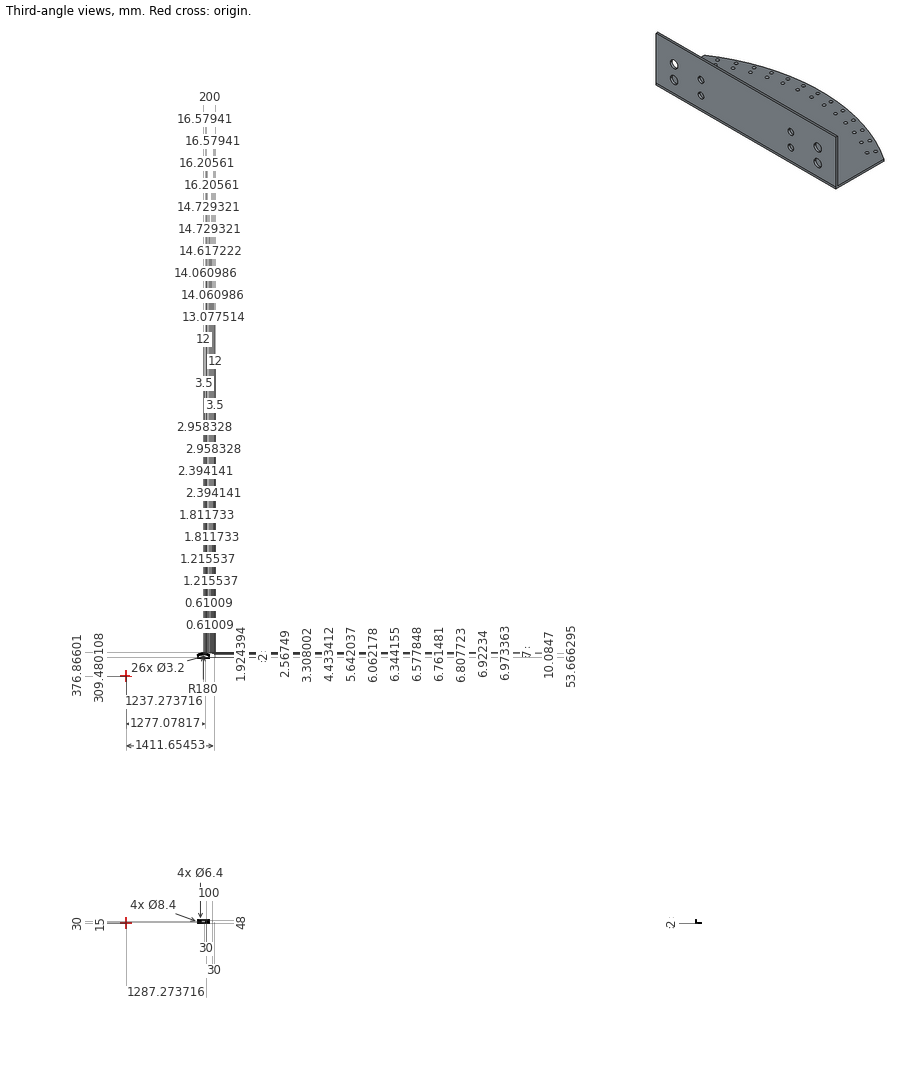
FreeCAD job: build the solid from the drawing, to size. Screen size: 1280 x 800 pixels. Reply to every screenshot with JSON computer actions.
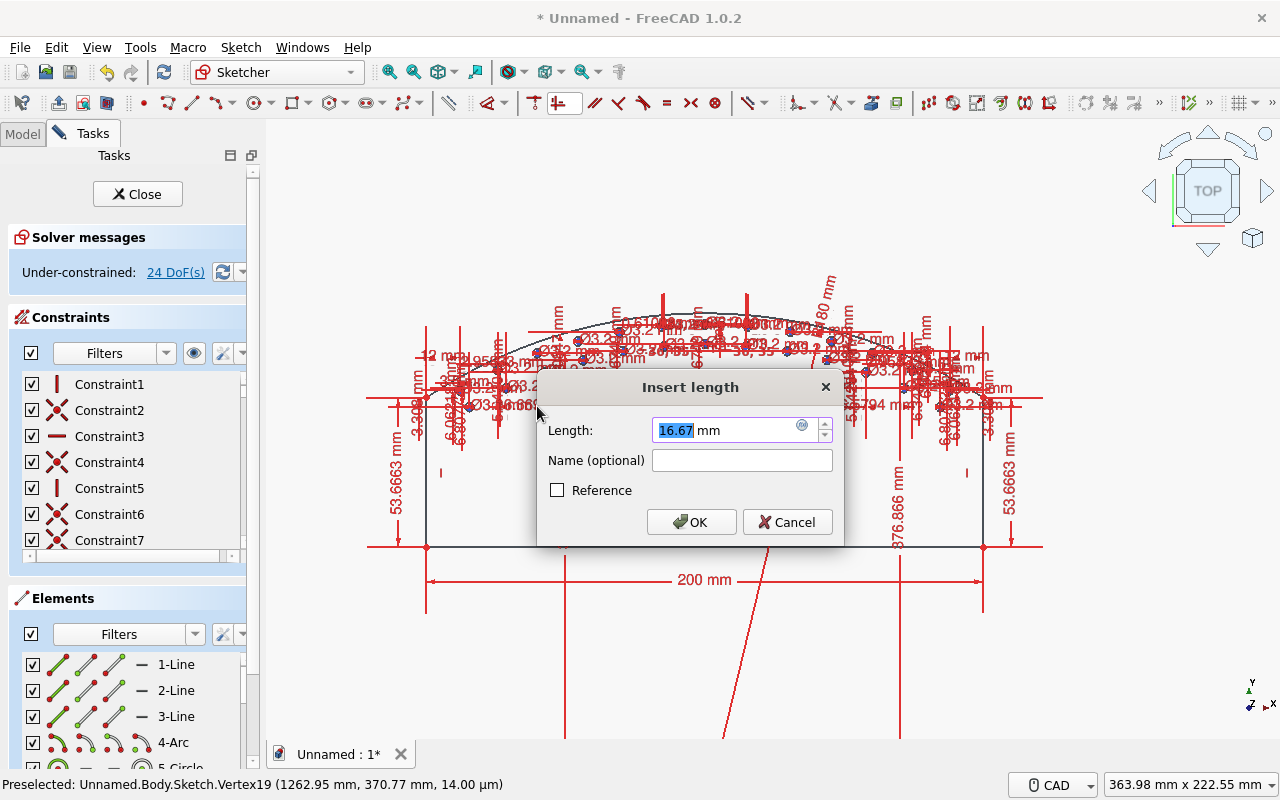
{"action": "type", "text": "16.57941"}
{"action": "key", "text": "Return"}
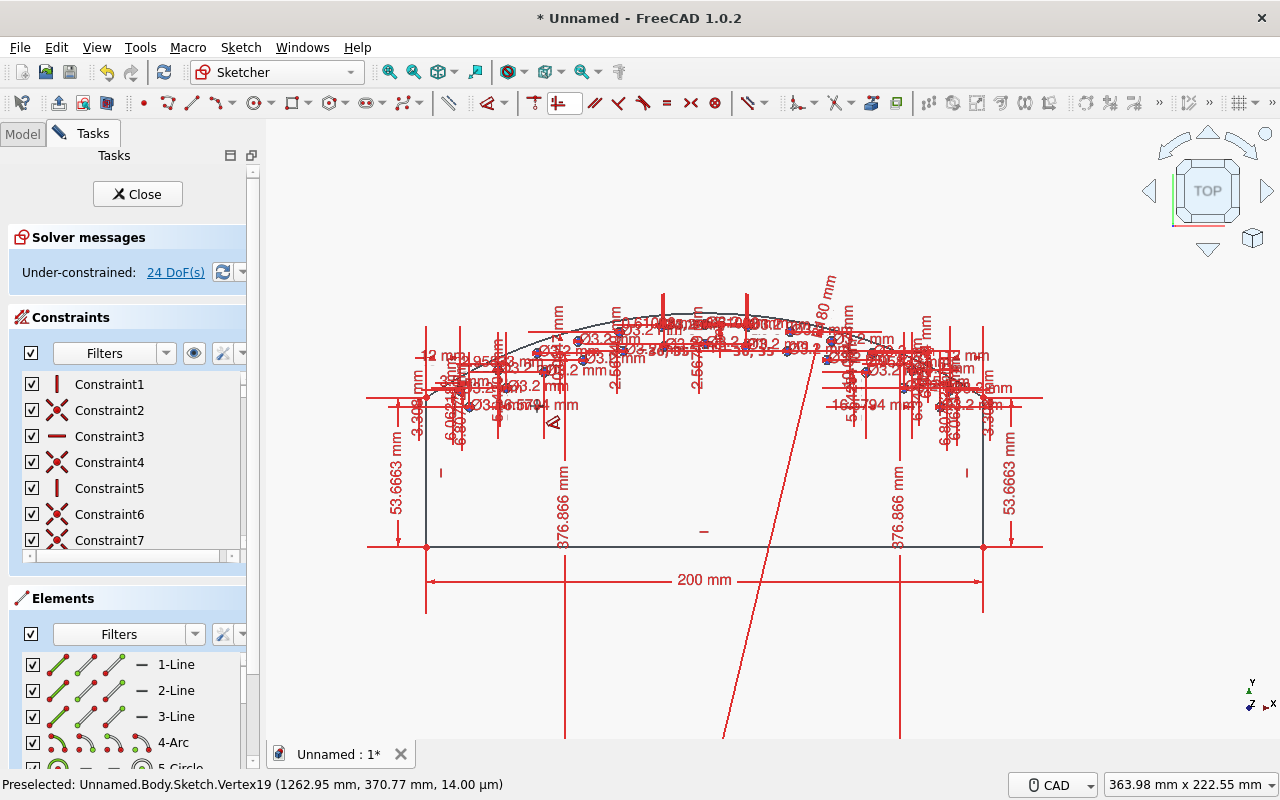
{"action": "scroll", "coordinate": [506, 388], "scroll_direction": "up", "scroll_amount": 5}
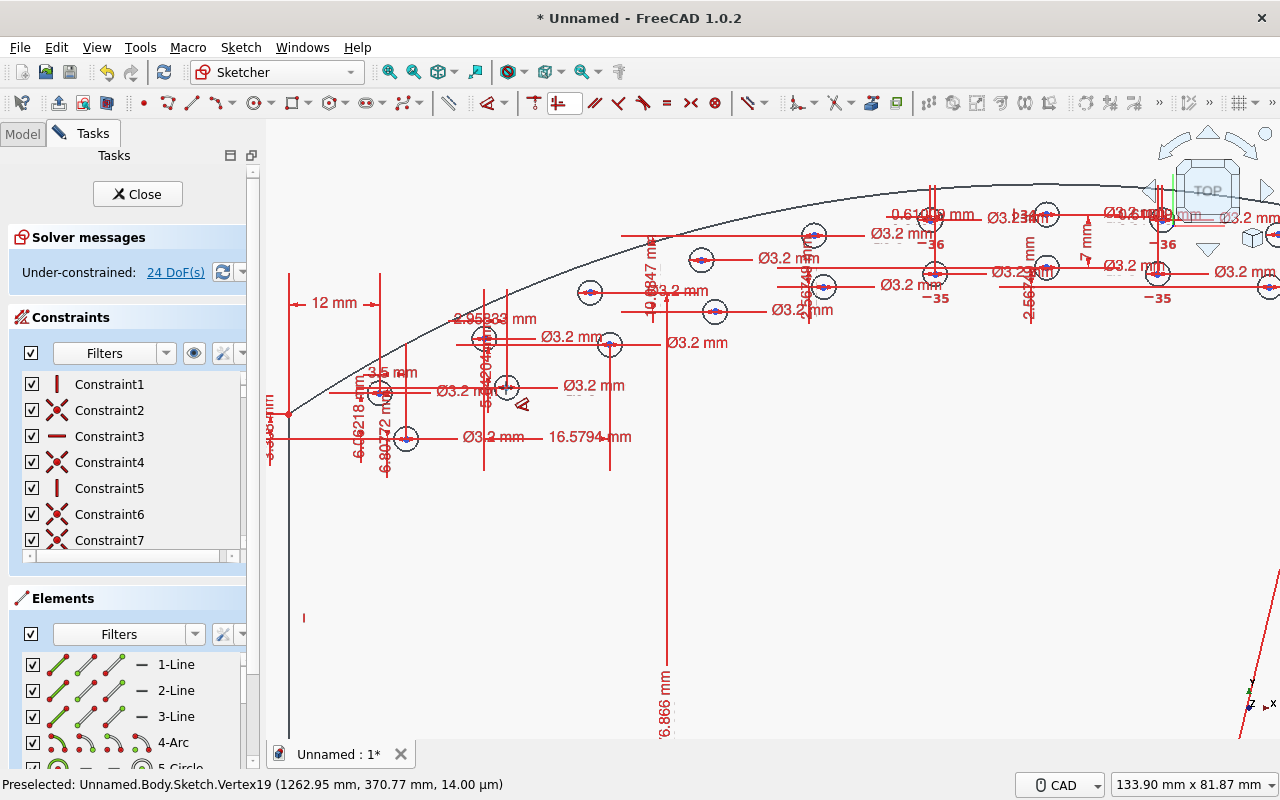
{"action": "left_click", "coordinate": [507, 388]}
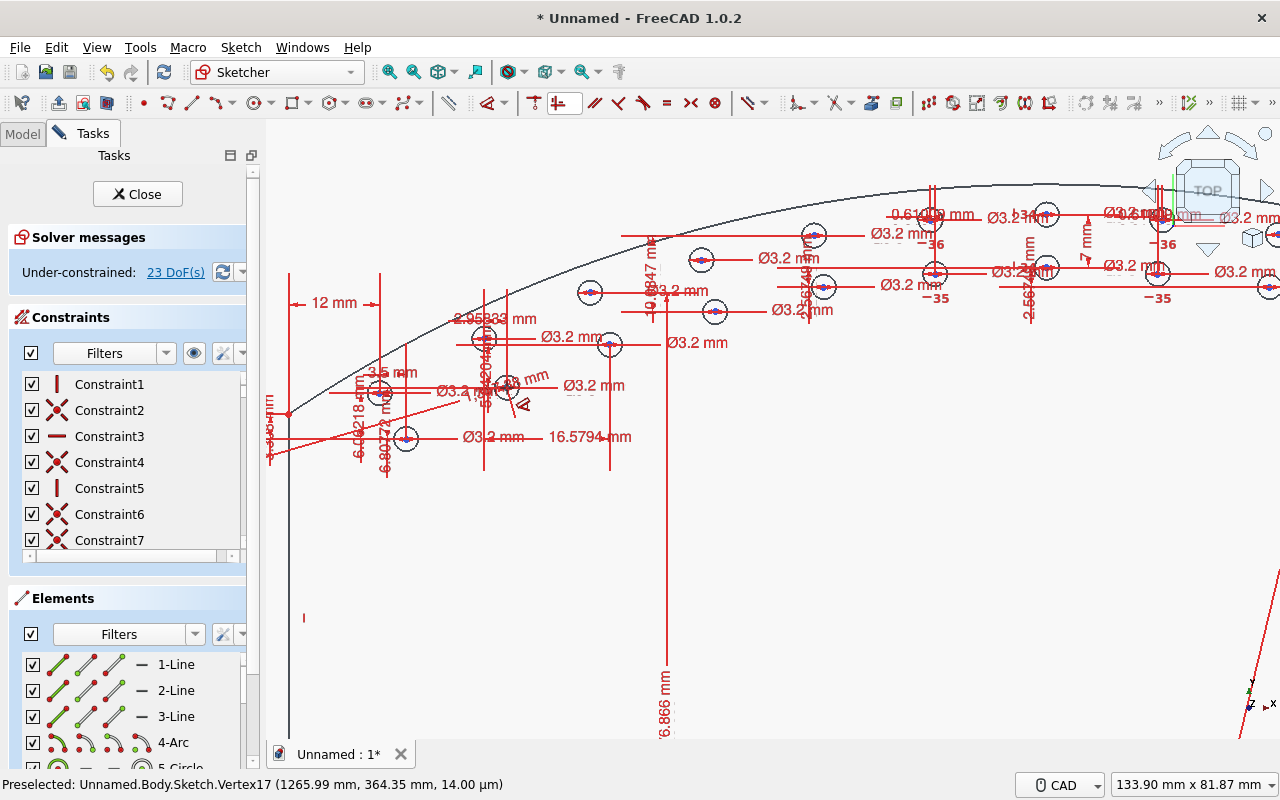
{"action": "left_click", "coordinate": [484, 339]}
{"action": "left_click", "coordinate": [450, 346]}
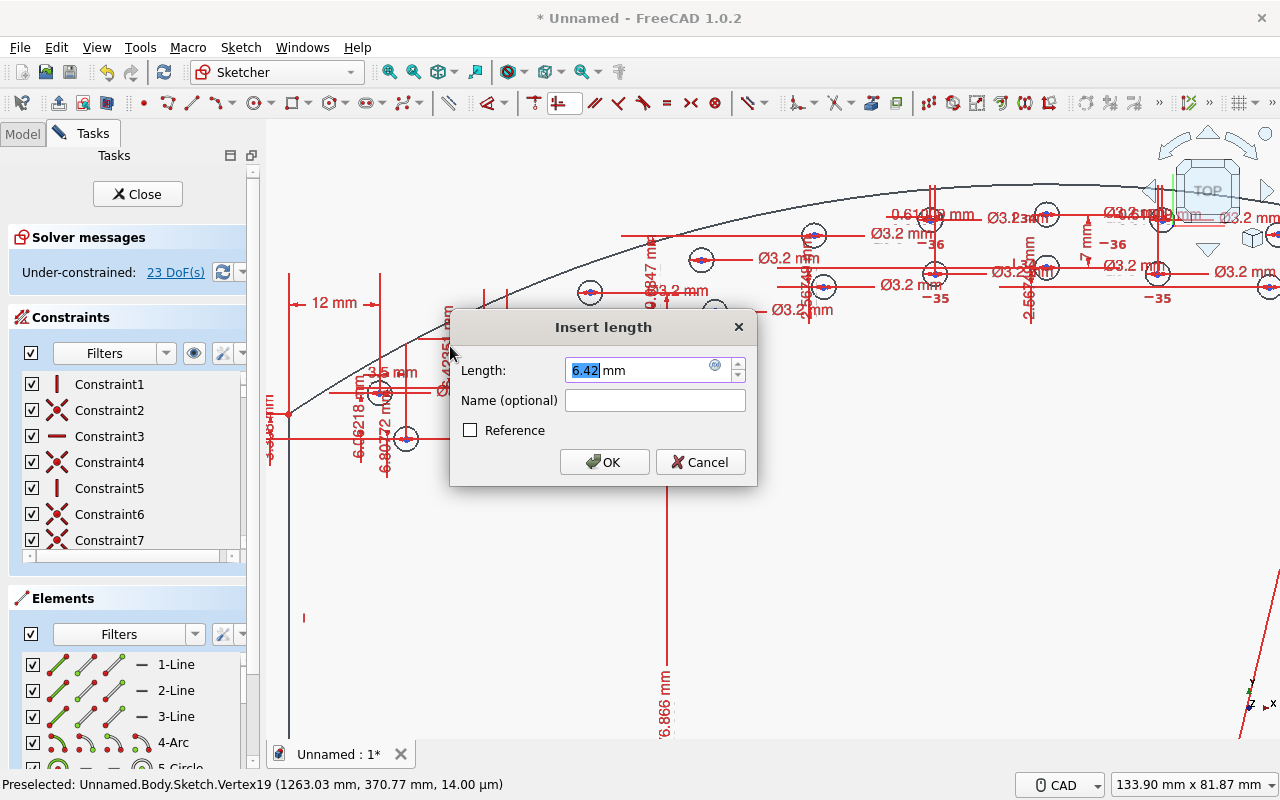
{"action": "type", "text": "6.344155"}
{"action": "key", "text": "Return"}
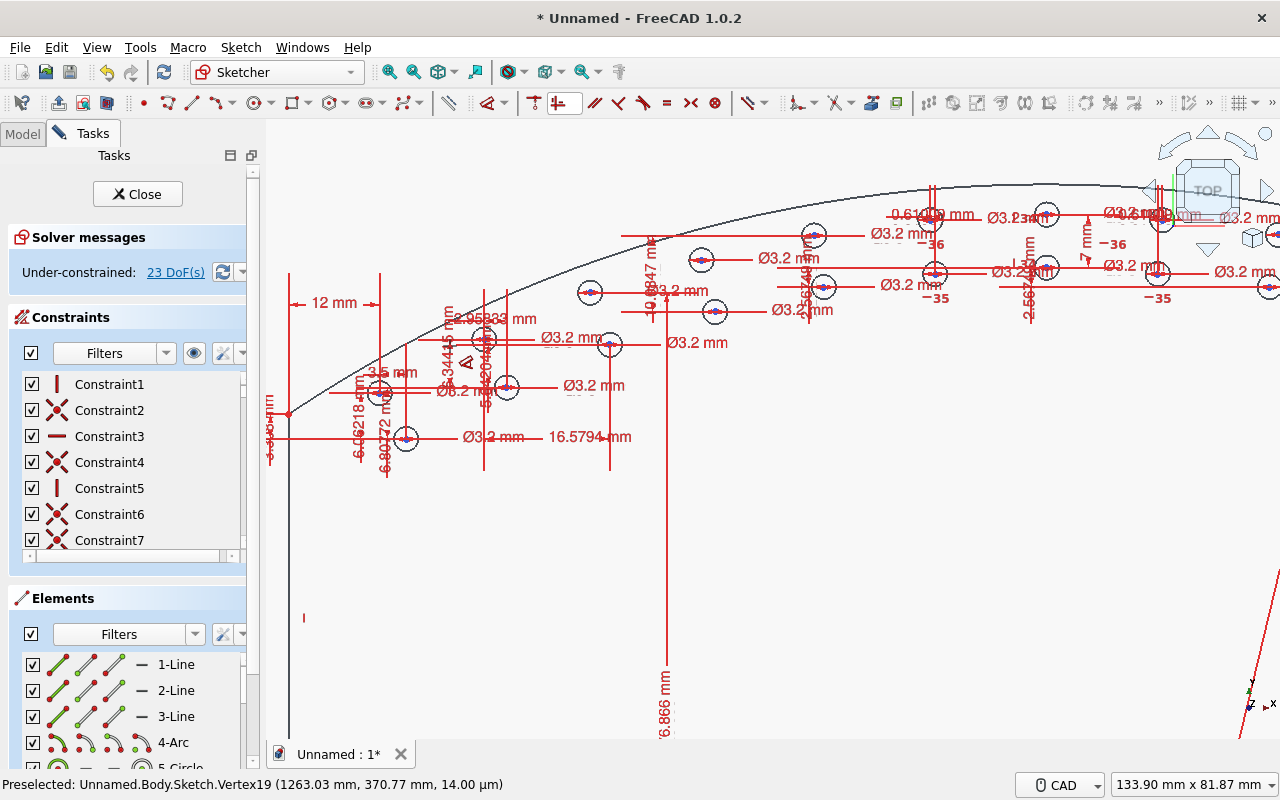
{"action": "scroll", "coordinate": [505, 388], "scroll_direction": "down", "scroll_amount": 5}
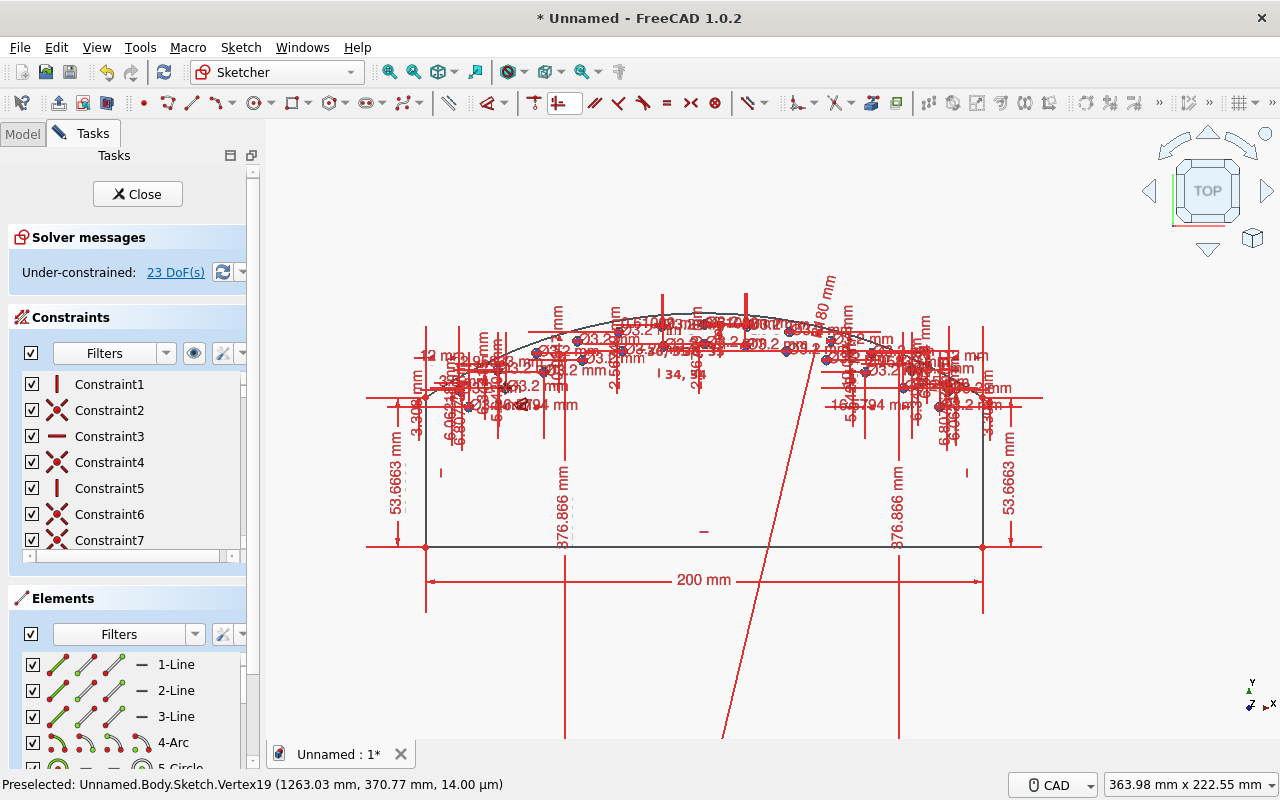
{"action": "scroll", "coordinate": [865, 372], "scroll_direction": "up", "scroll_amount": 9}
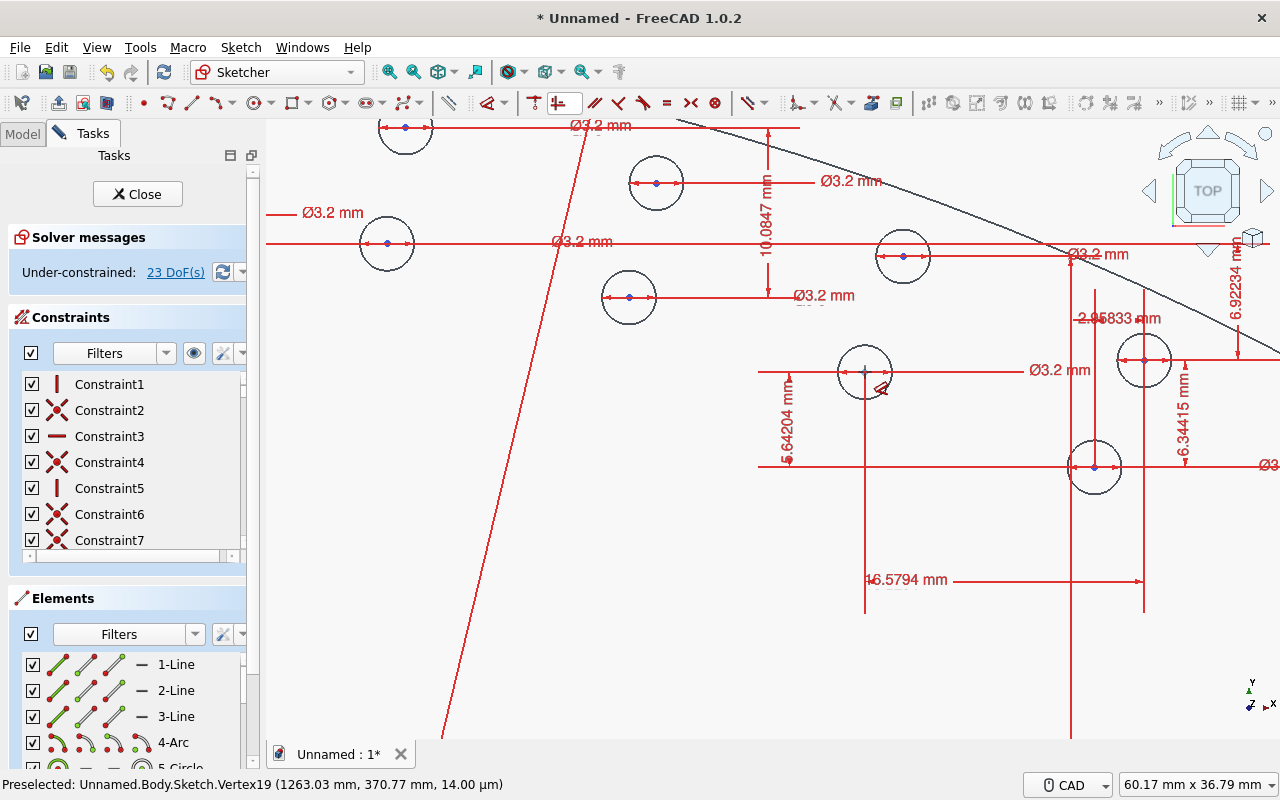
{"action": "left_click", "coordinate": [865, 372]}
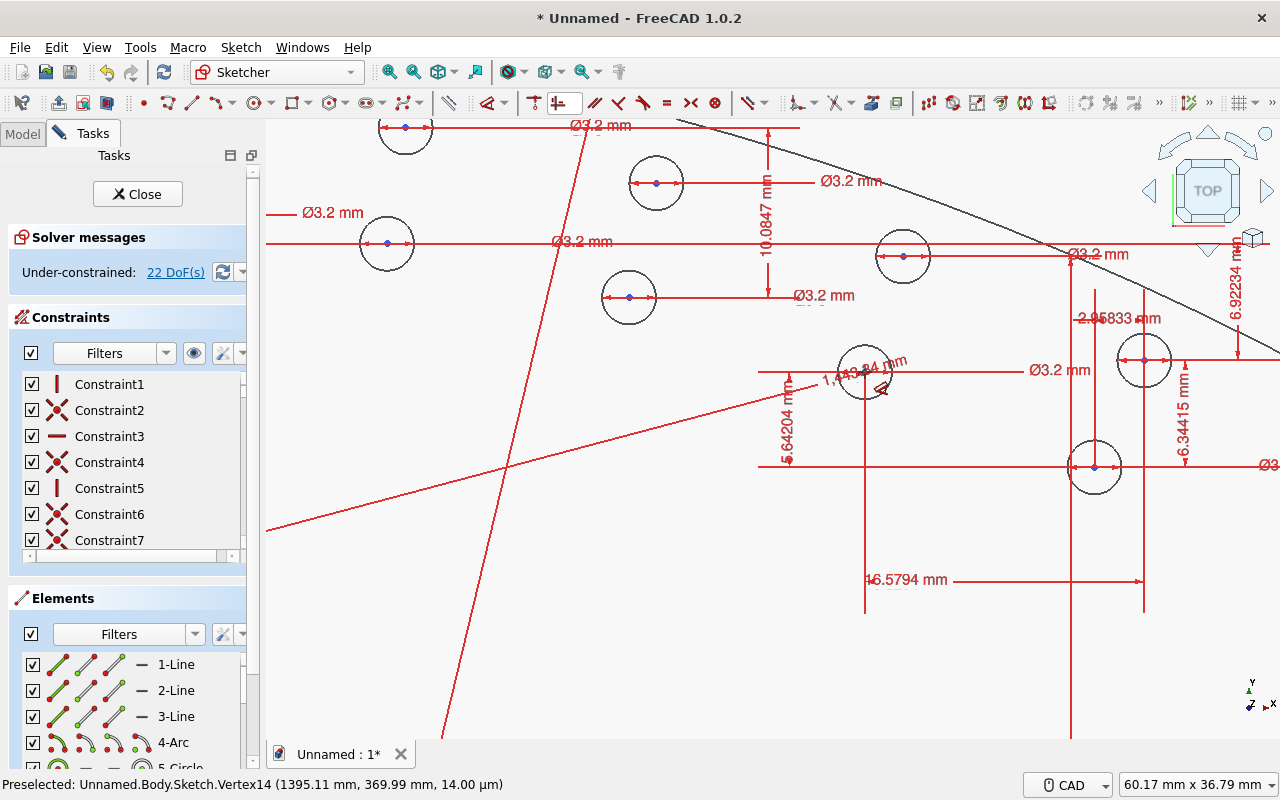
{"action": "left_click", "coordinate": [903, 256]}
{"action": "left_click", "coordinate": [875, 222]}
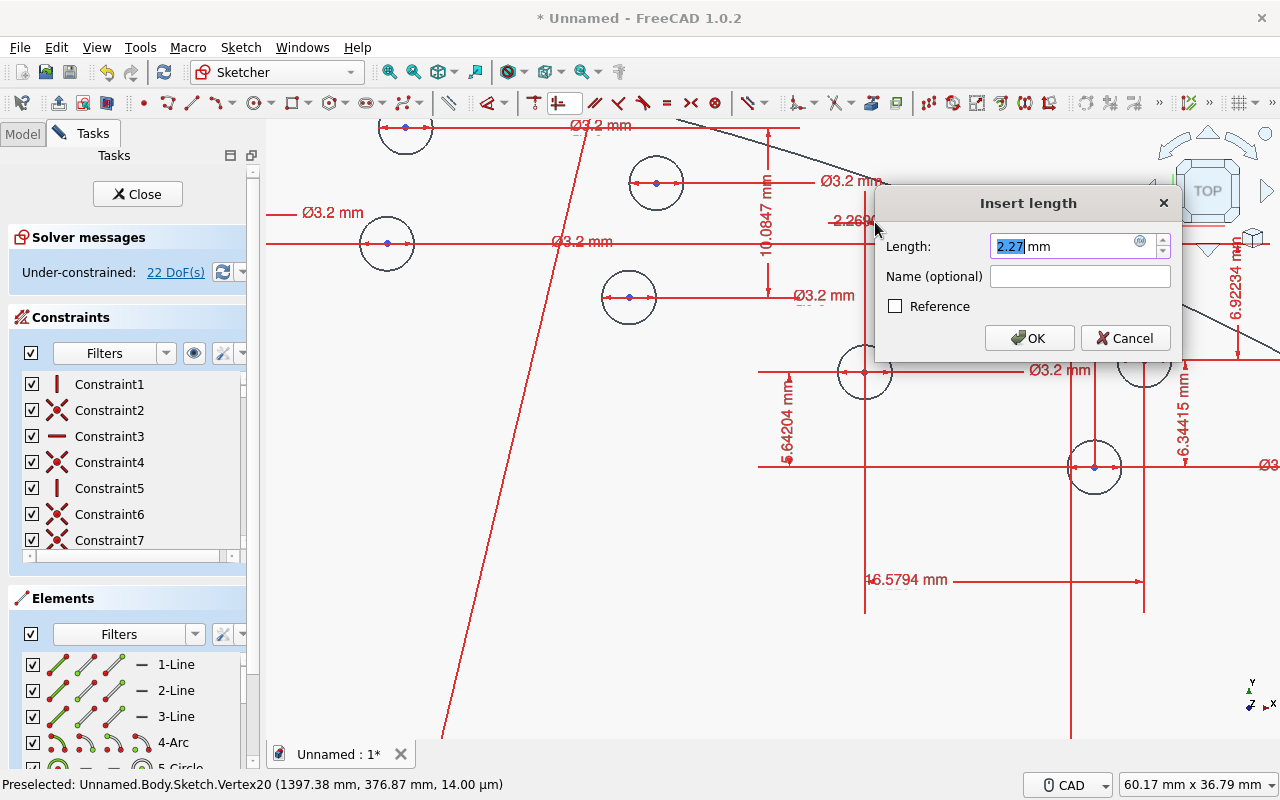
{"action": "type", "text": "2.394141"}
{"action": "key", "text": "Return"}